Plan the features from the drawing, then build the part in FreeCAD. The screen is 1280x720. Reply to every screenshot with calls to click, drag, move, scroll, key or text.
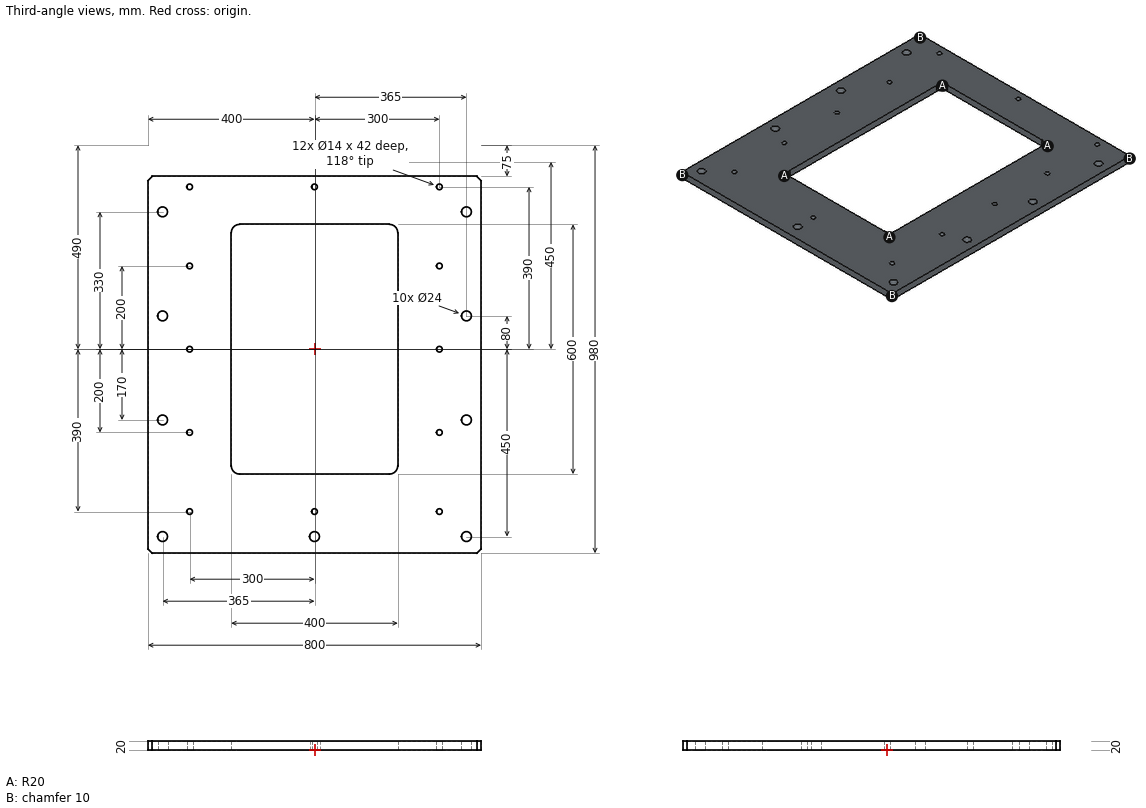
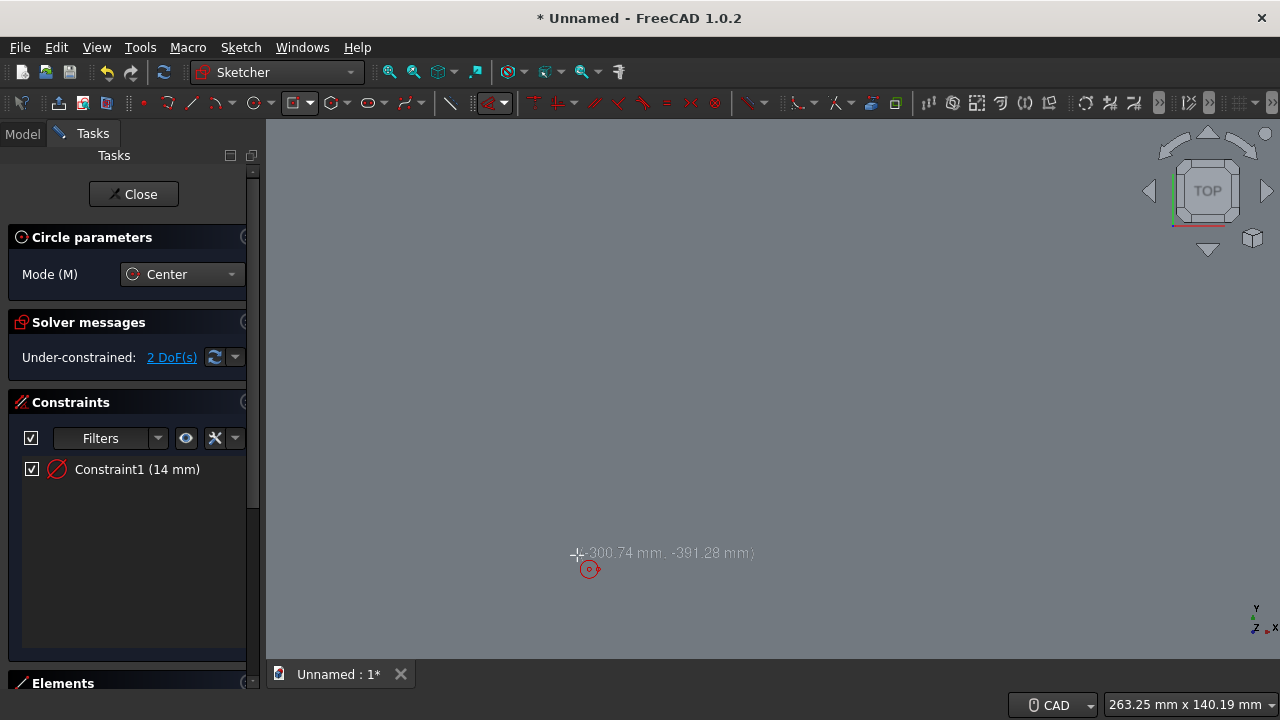
scroll(576, 556, down, 11)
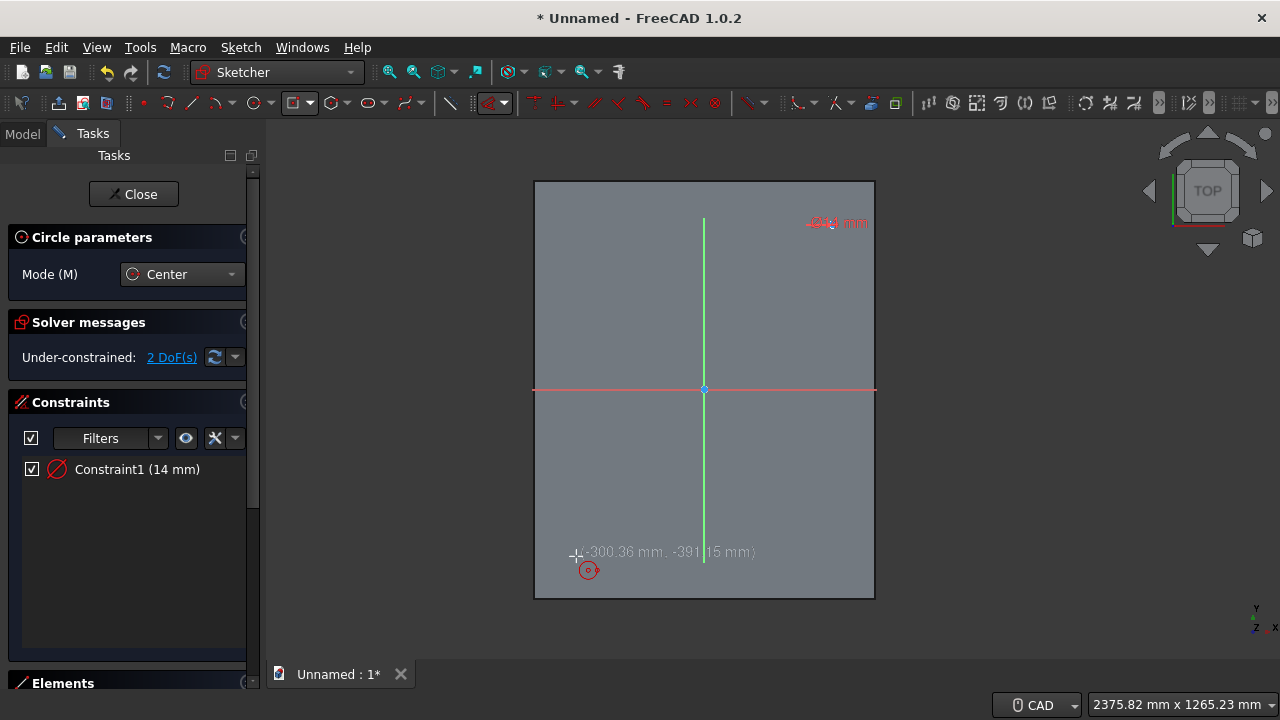
click(576, 556)
move(579, 554)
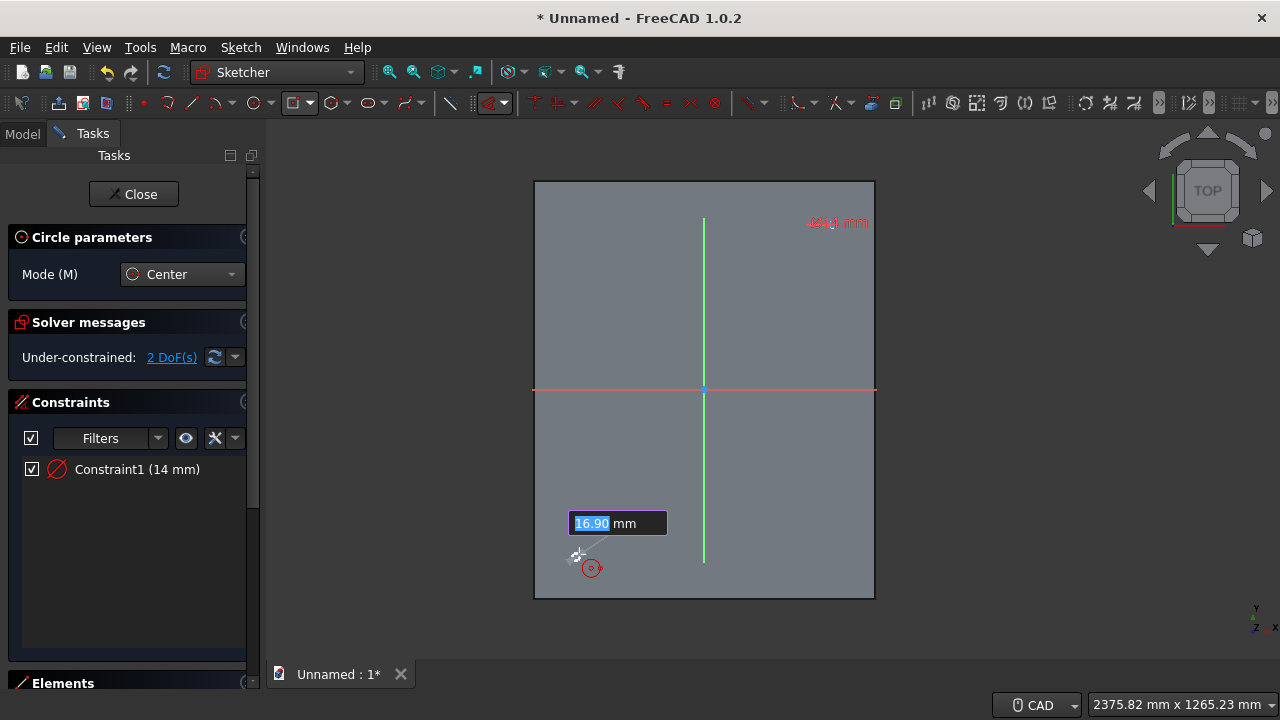
text(14)
key(Return)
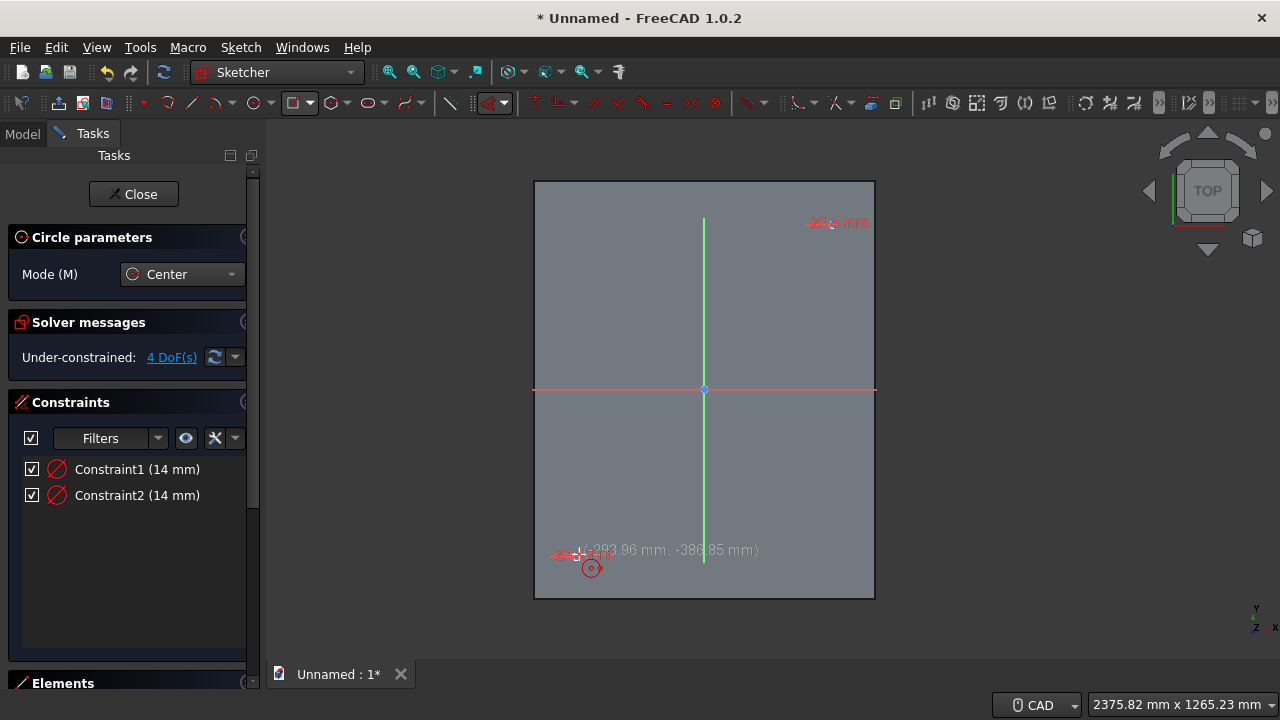
scroll(576, 223, up, 11)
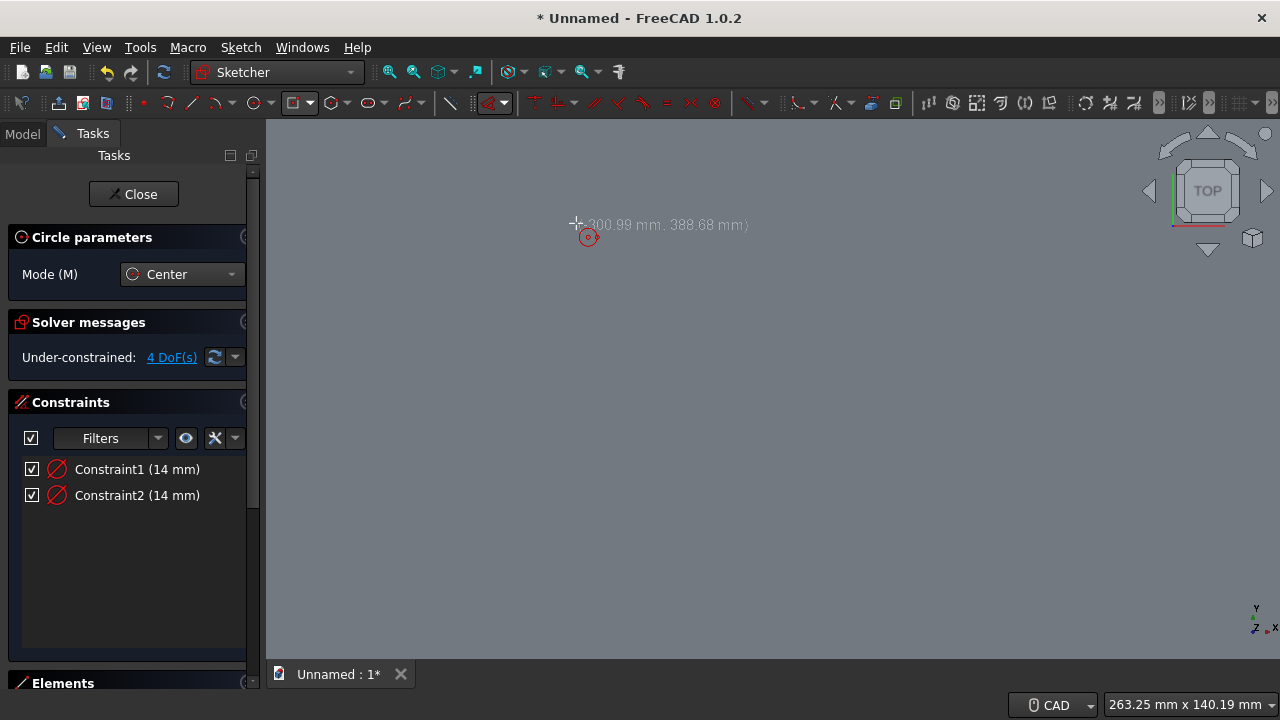
scroll(576, 222, down, 11)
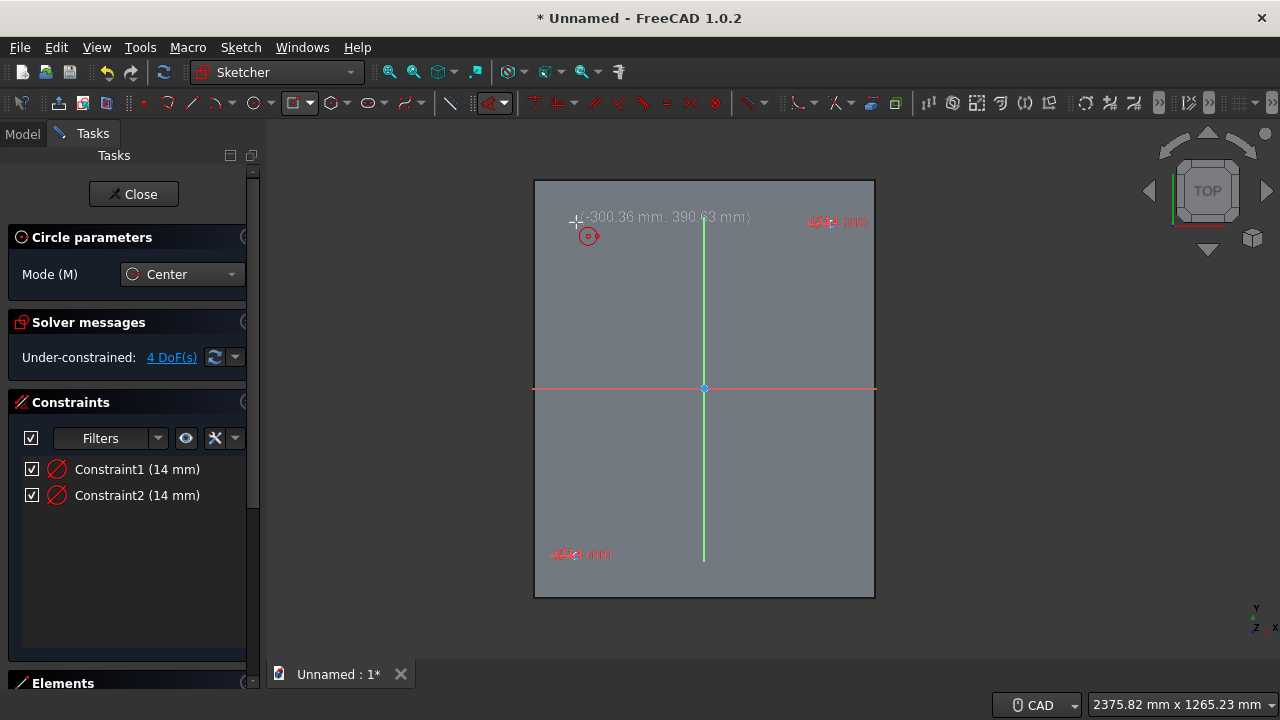
click(576, 223)
move(579, 220)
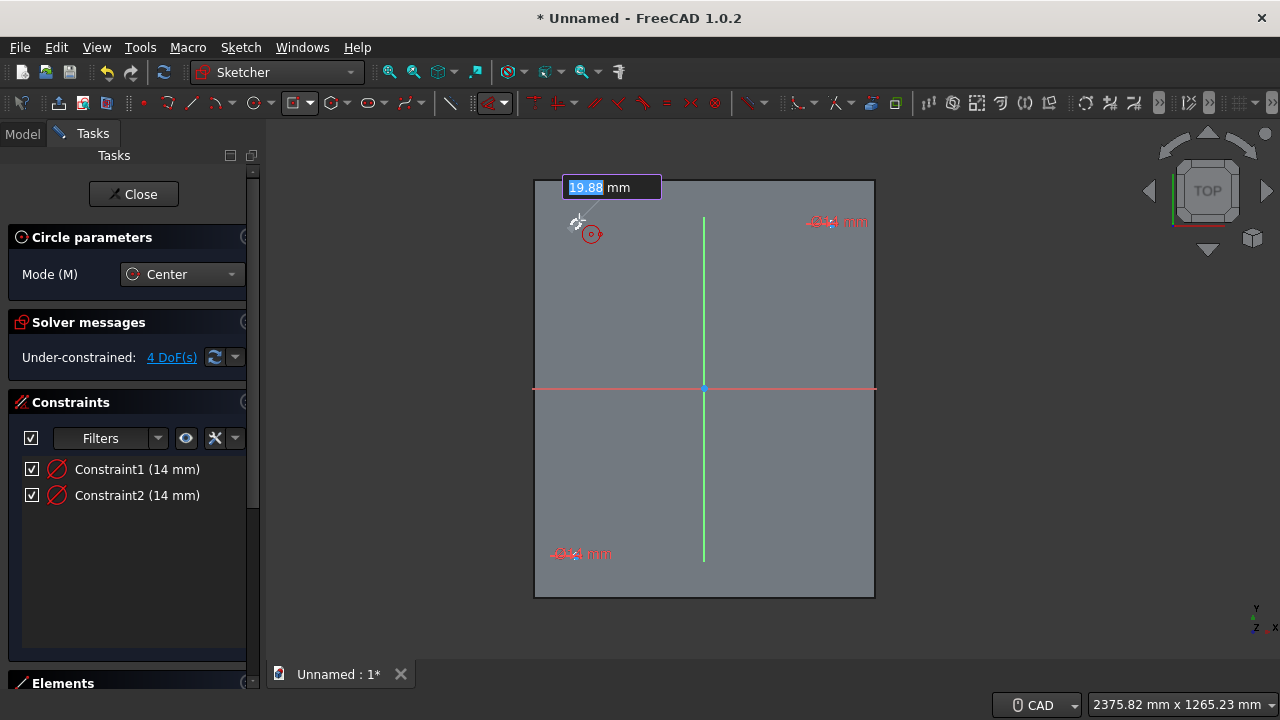
text(14)
key(Return)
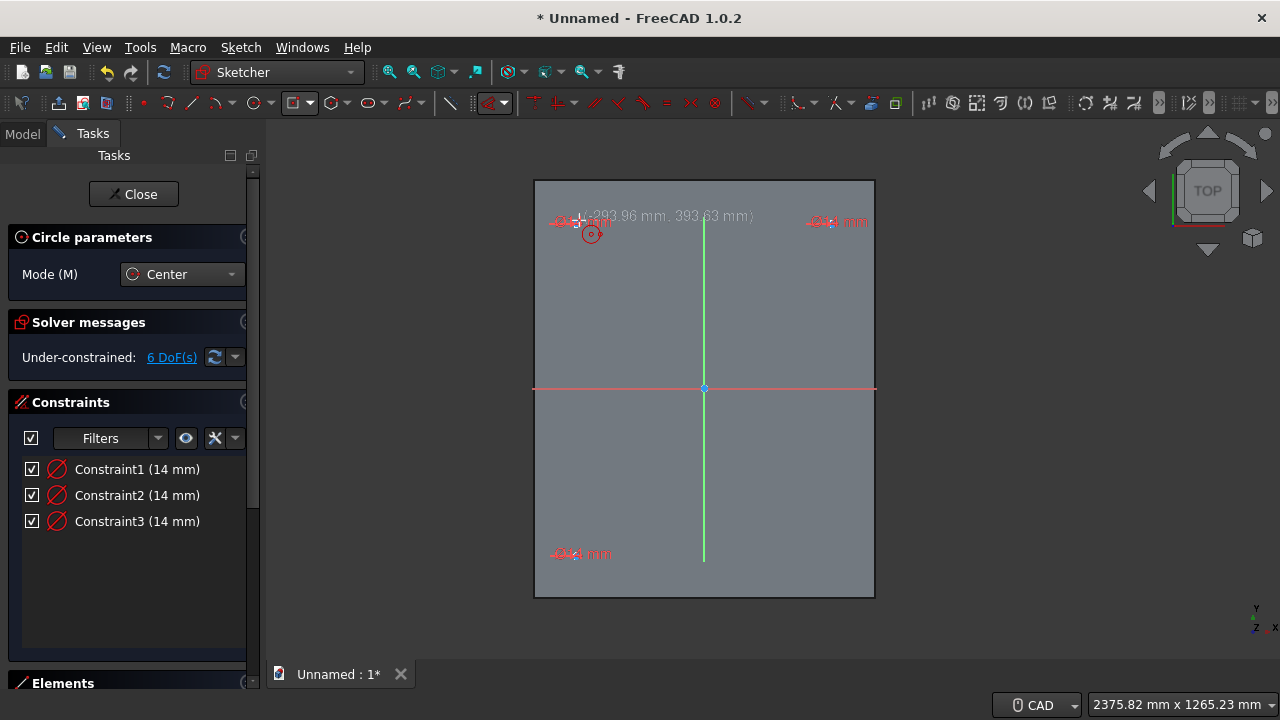
scroll(833, 555, up, 11)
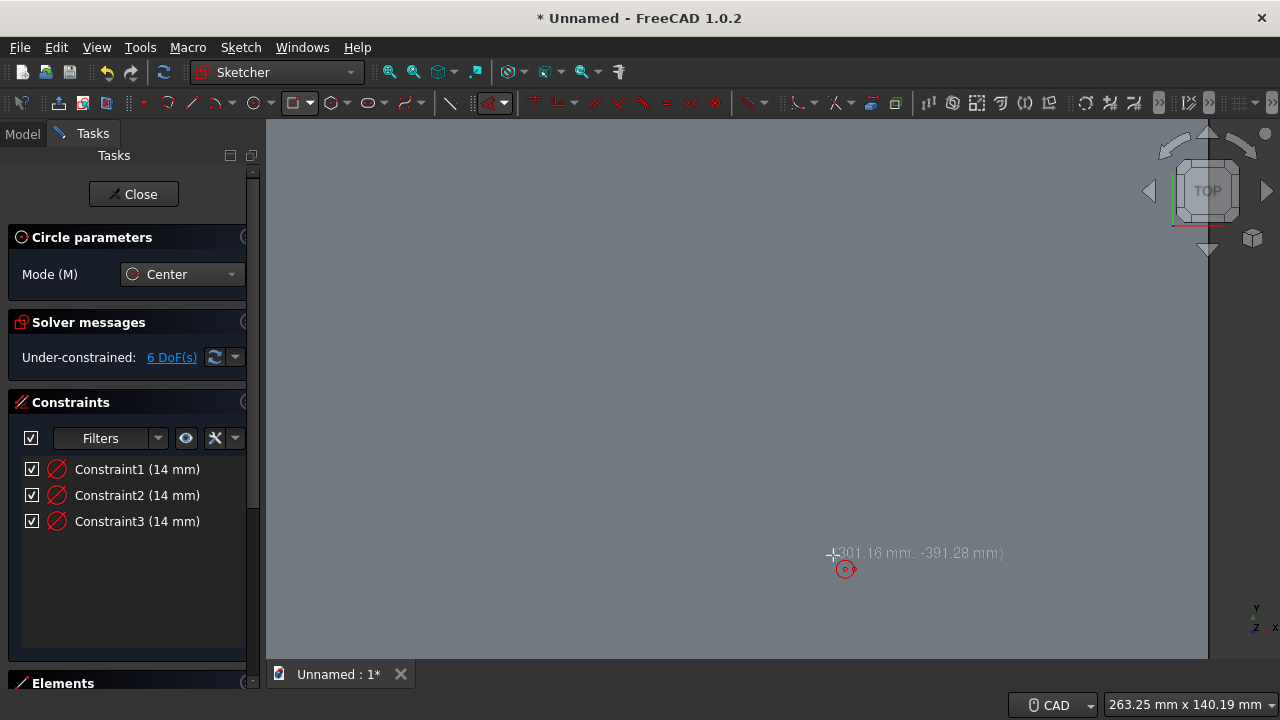
scroll(834, 556, down, 11)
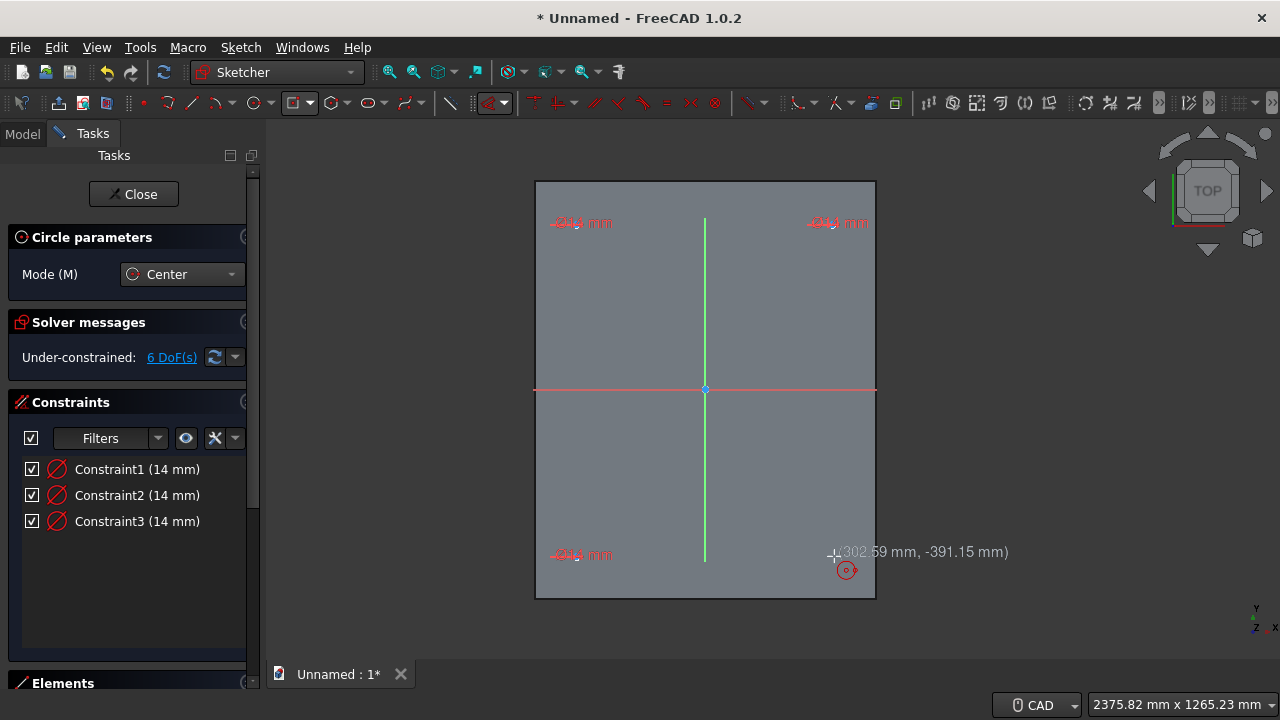
click(833, 556)
move(836, 554)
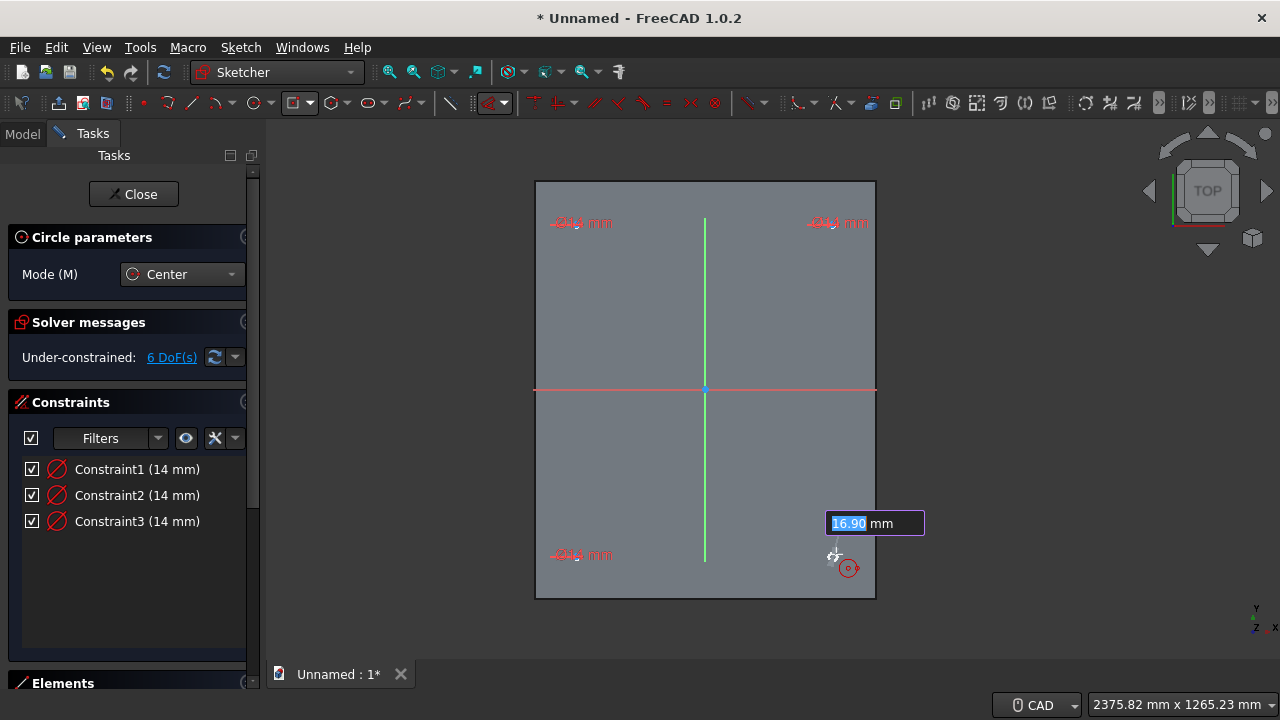
text(14)
key(Return)